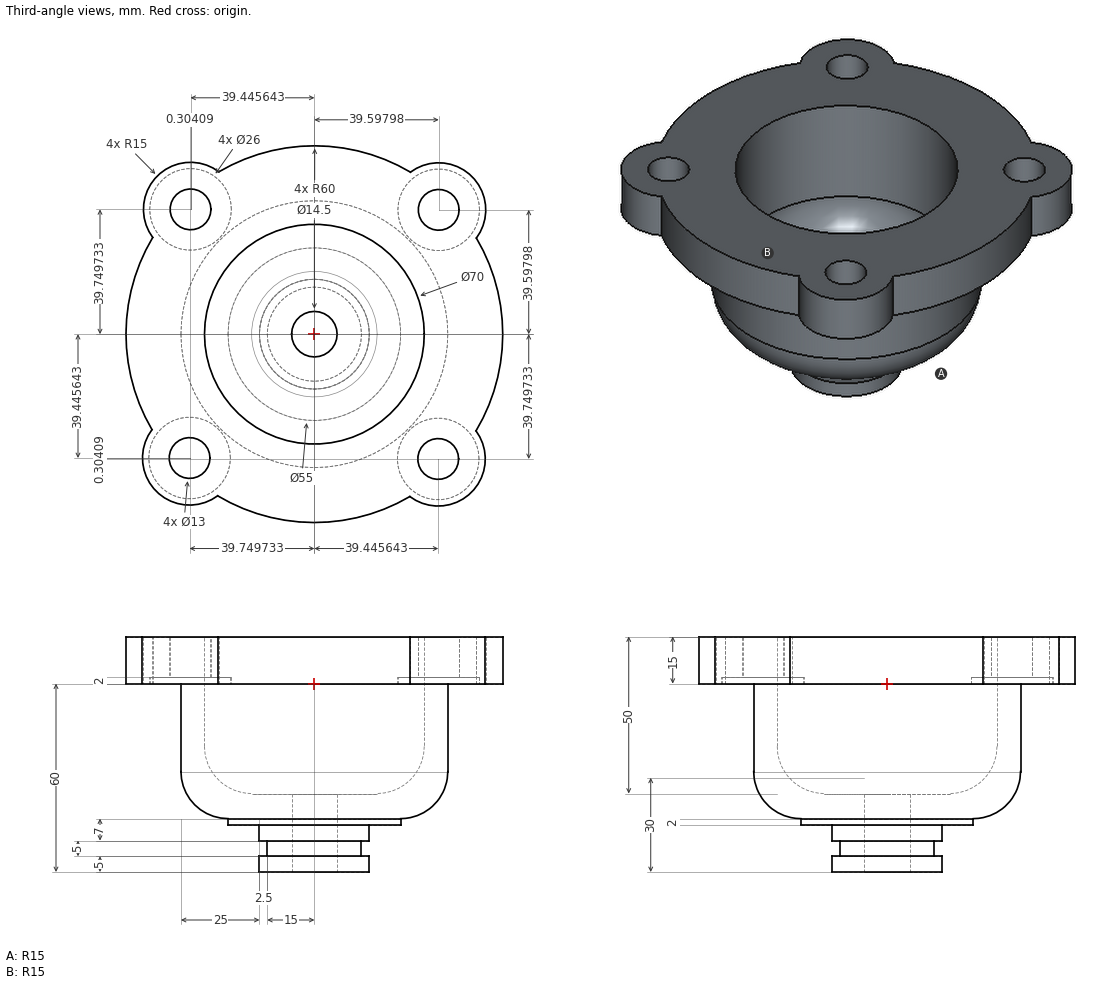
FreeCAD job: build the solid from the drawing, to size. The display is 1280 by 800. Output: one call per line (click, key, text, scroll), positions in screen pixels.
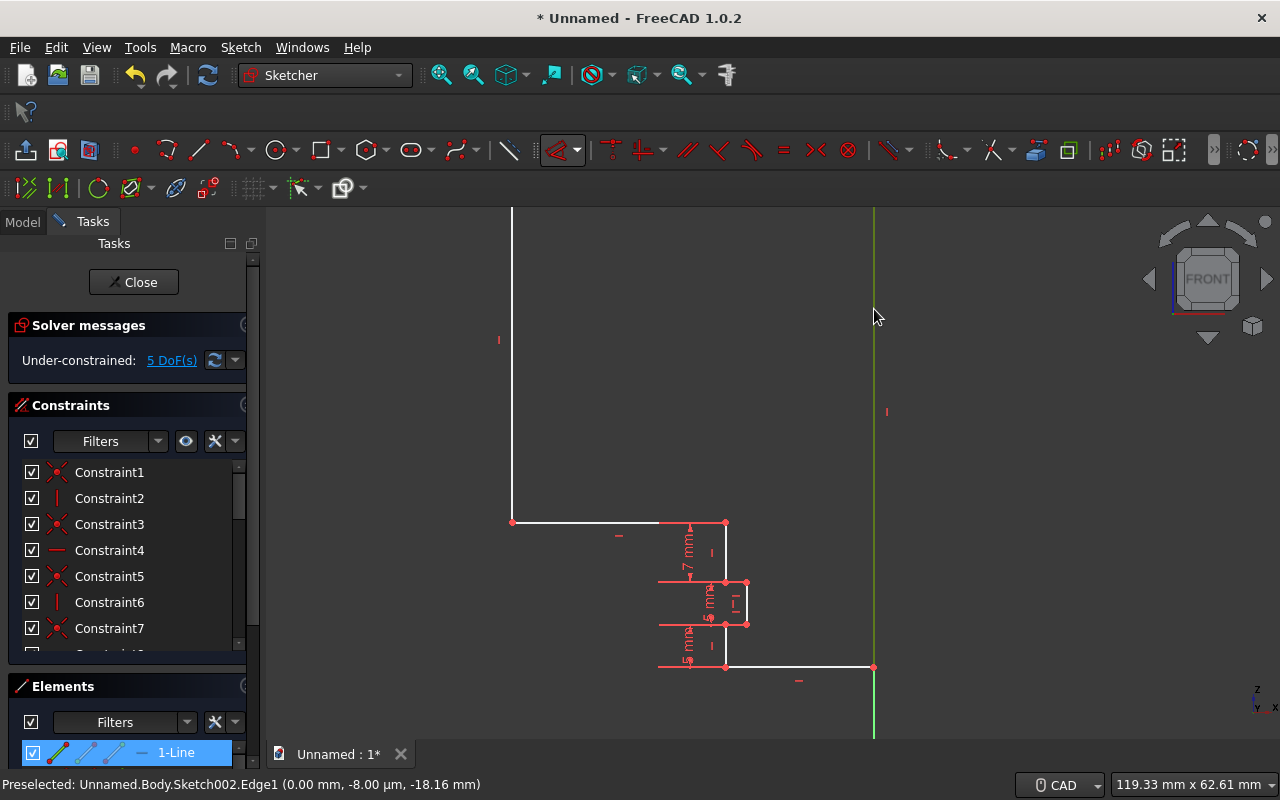
key(i)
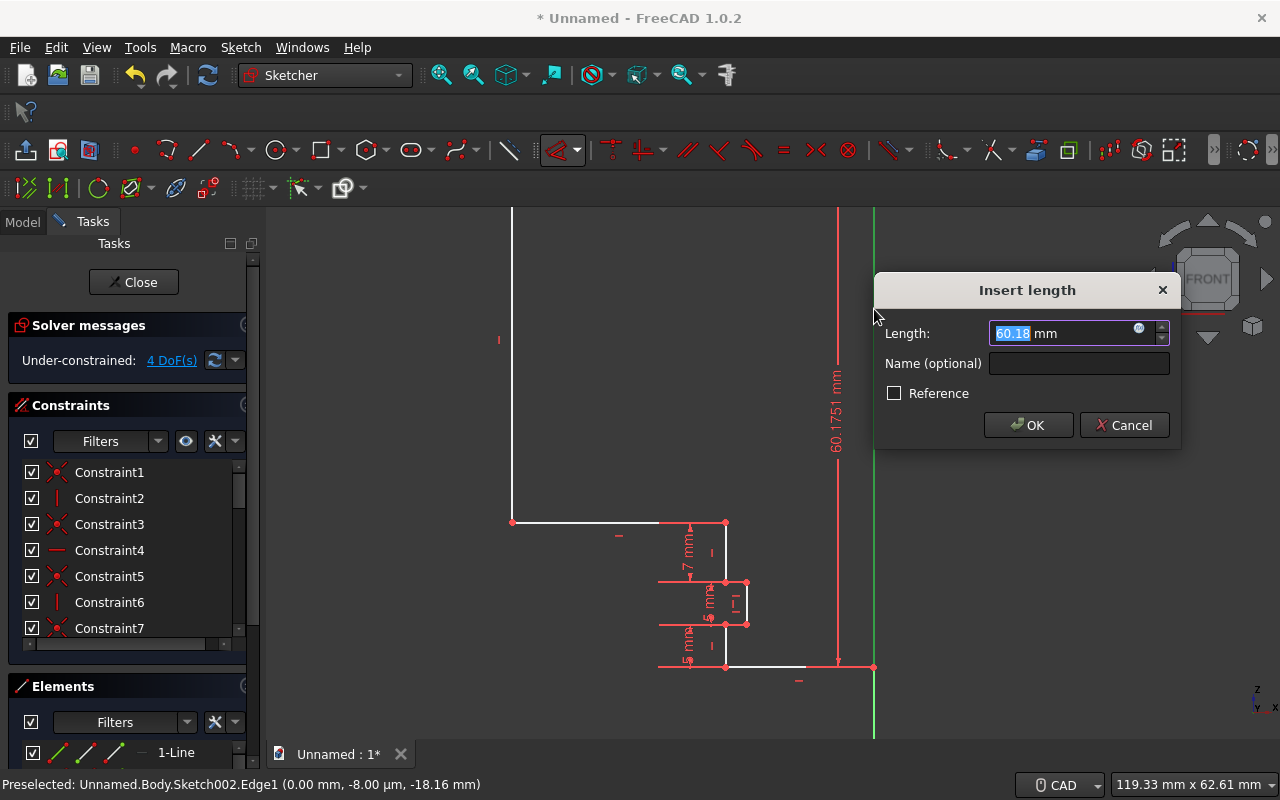
text(60)
key(Return)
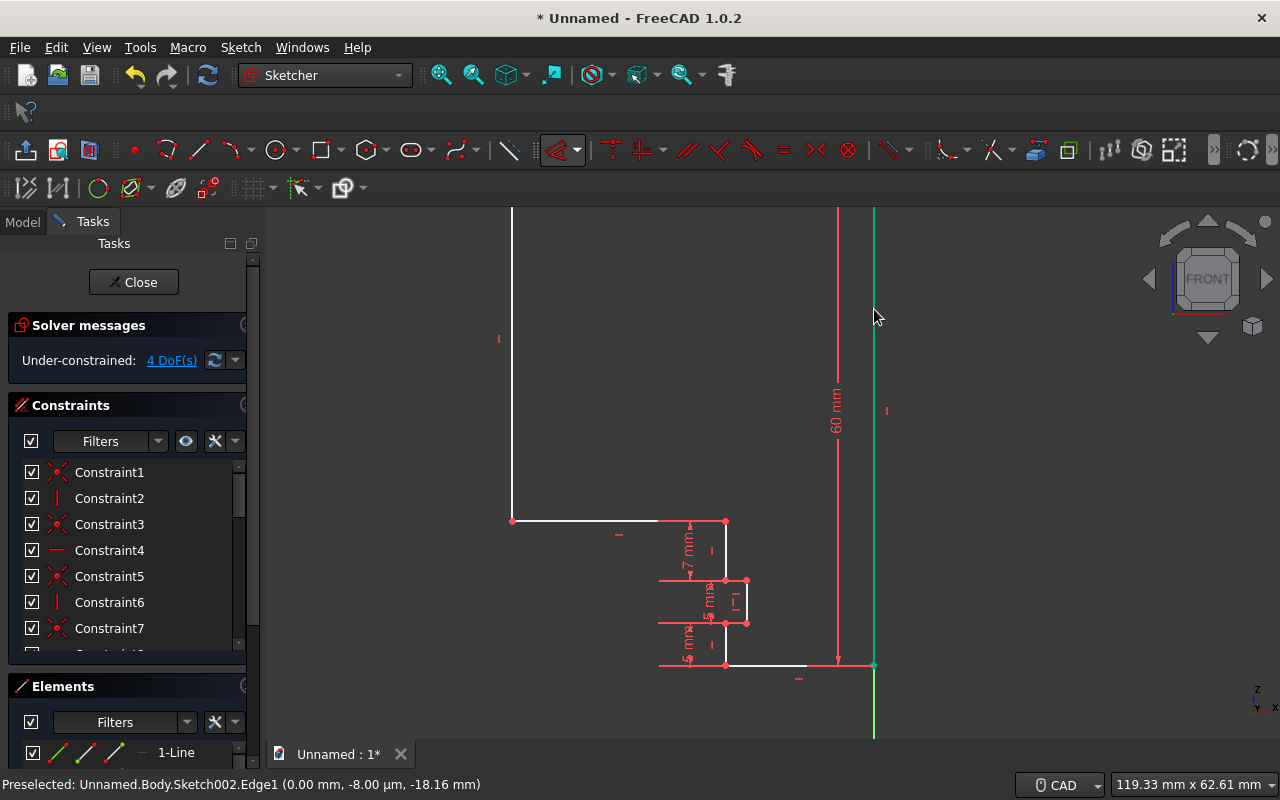
click(662, 521)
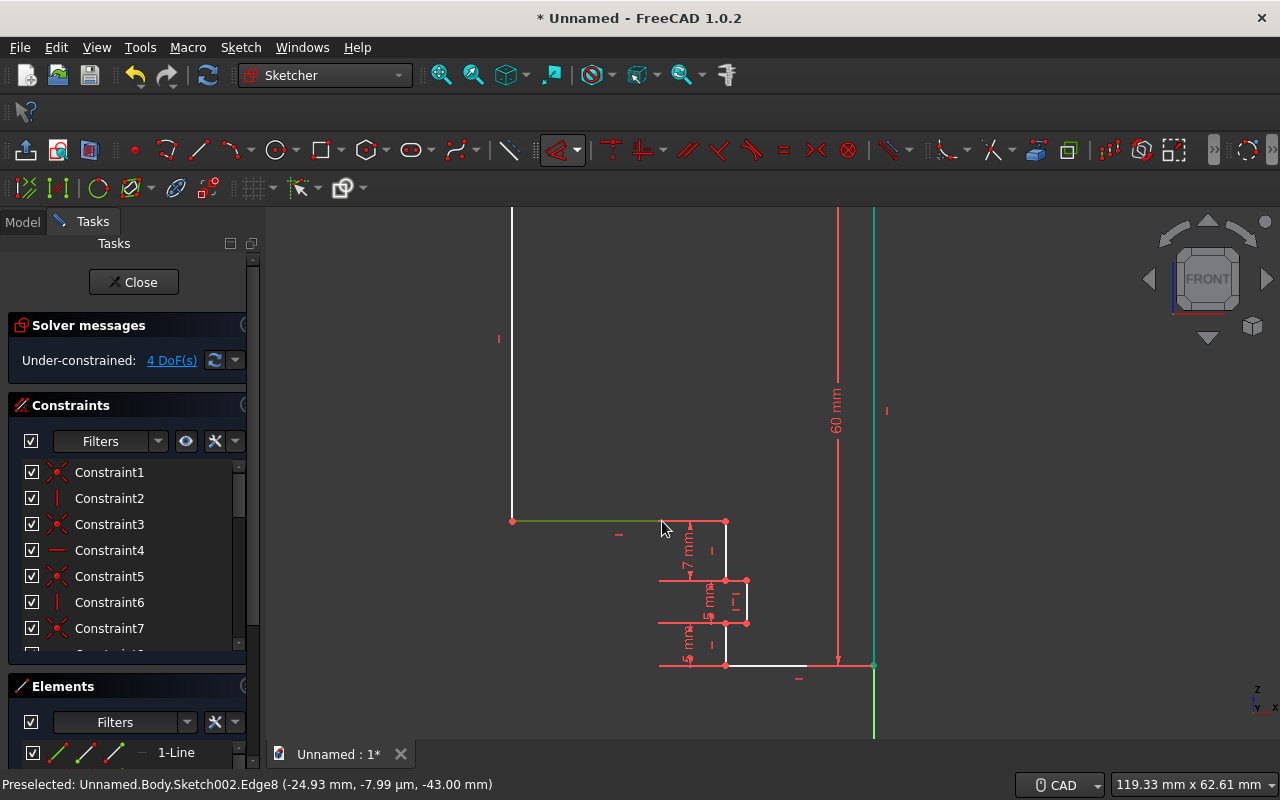
click(580, 150)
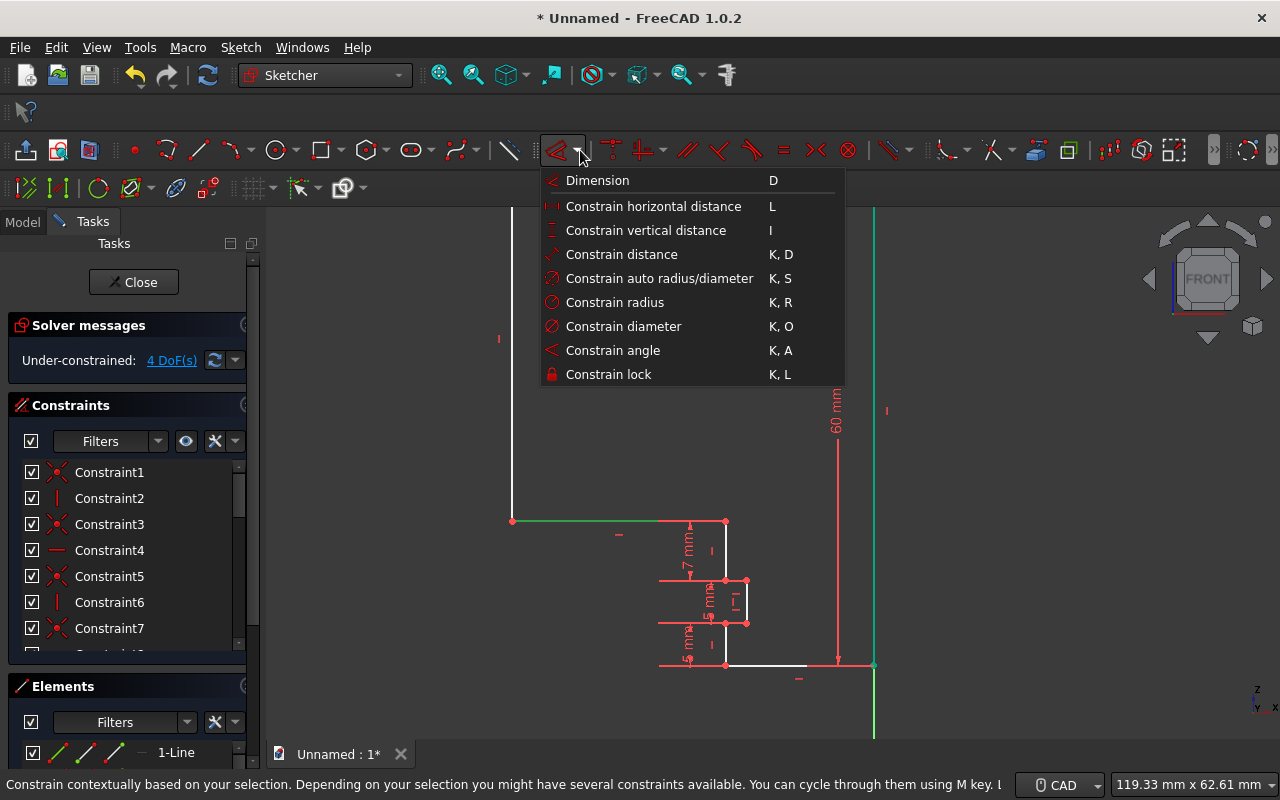
click(693, 206)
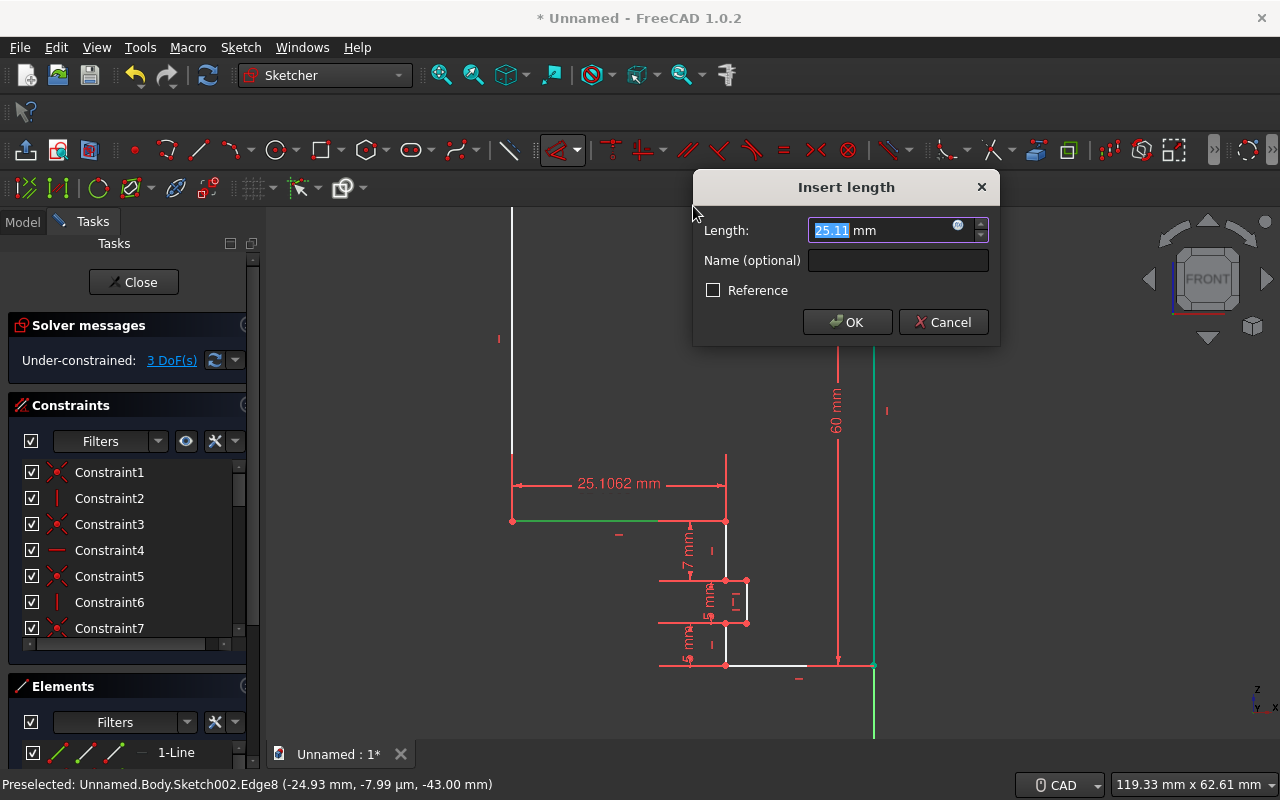
text(25)
key(Return)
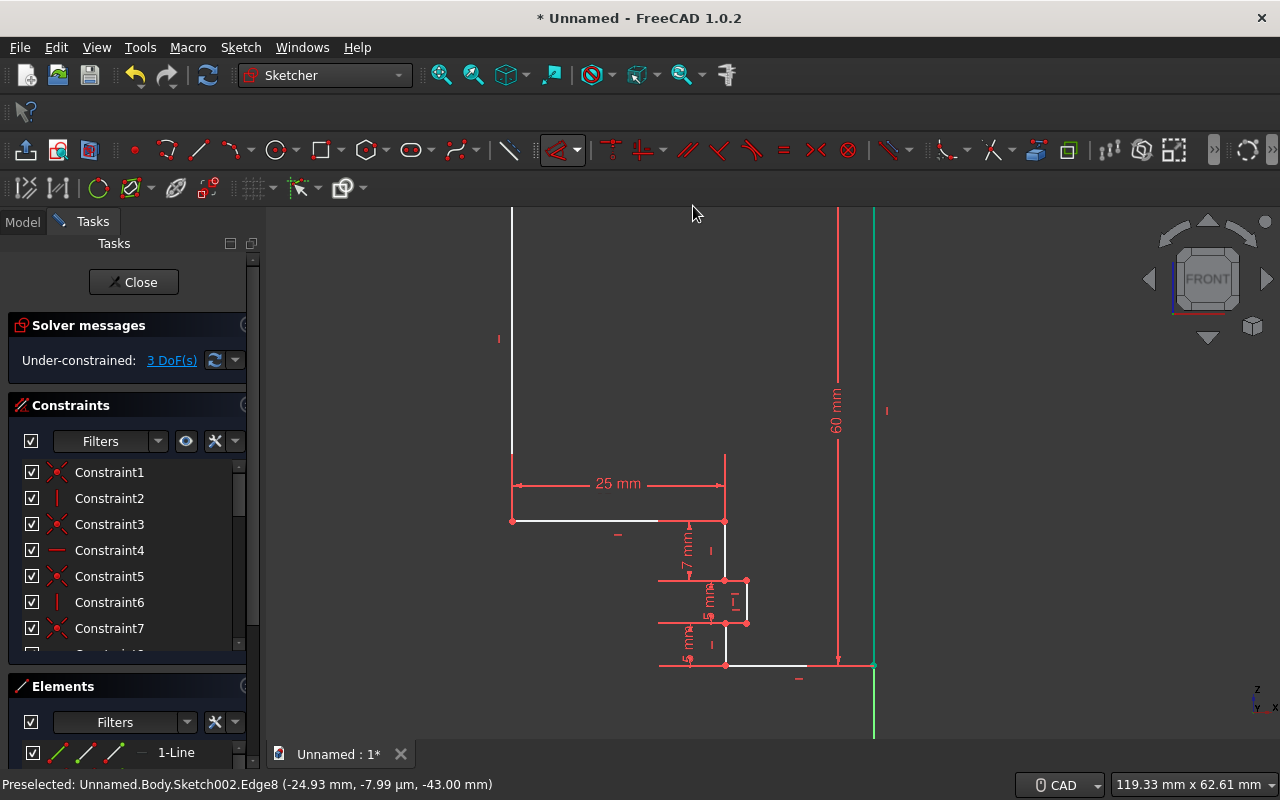
scroll(736, 623, up, 4)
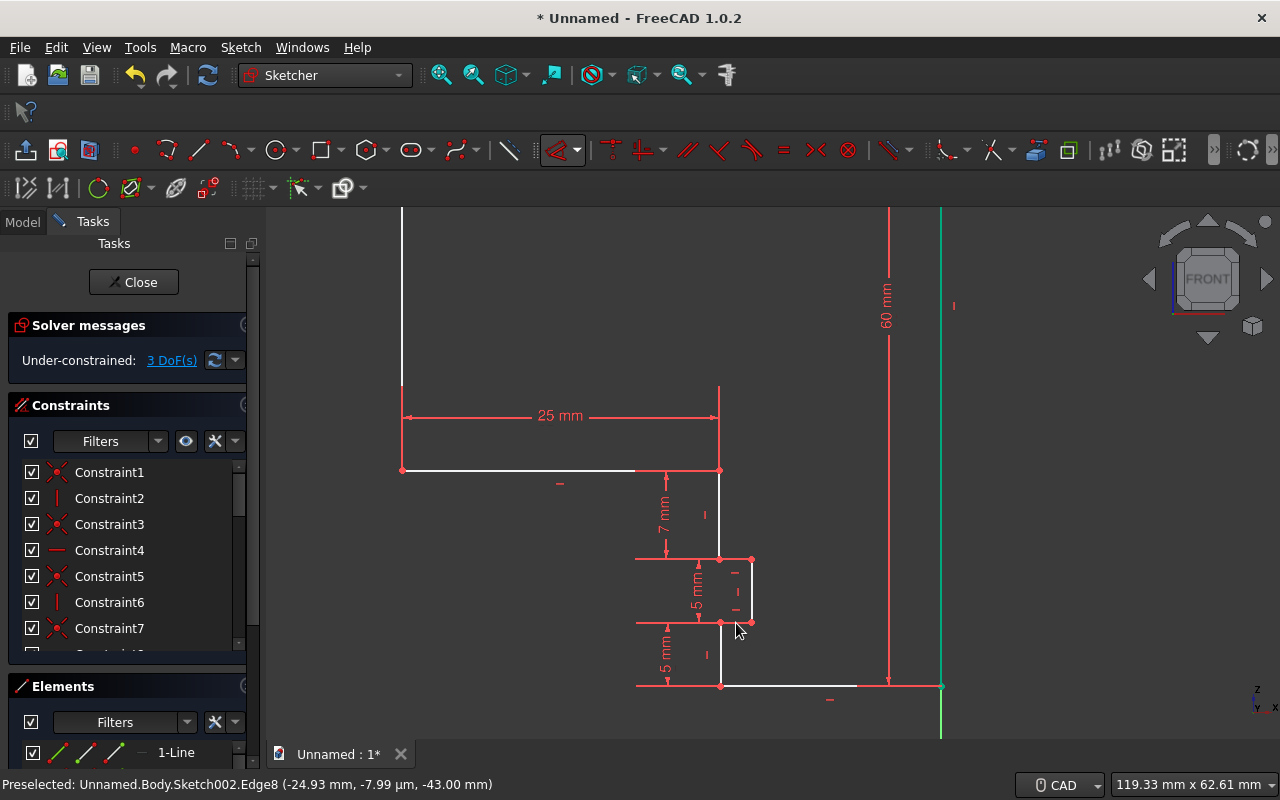
click(736, 622)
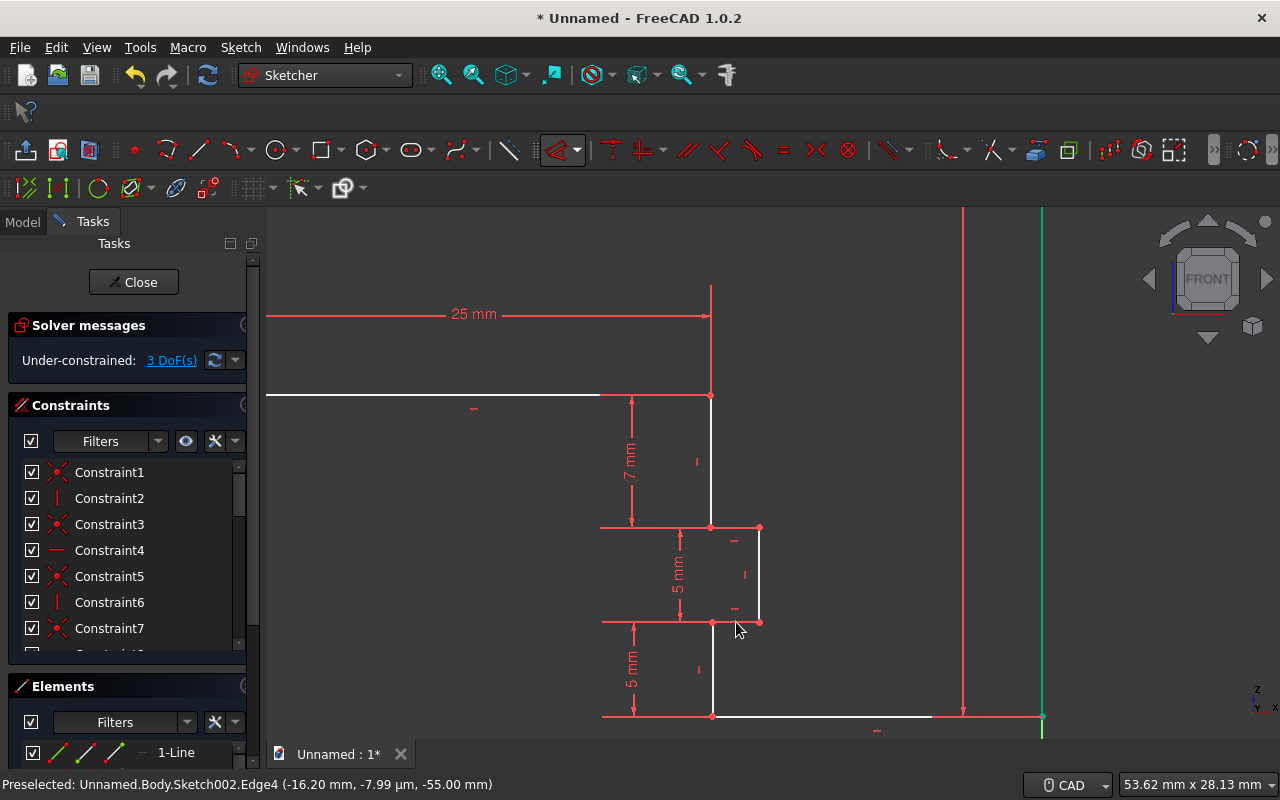
key(l)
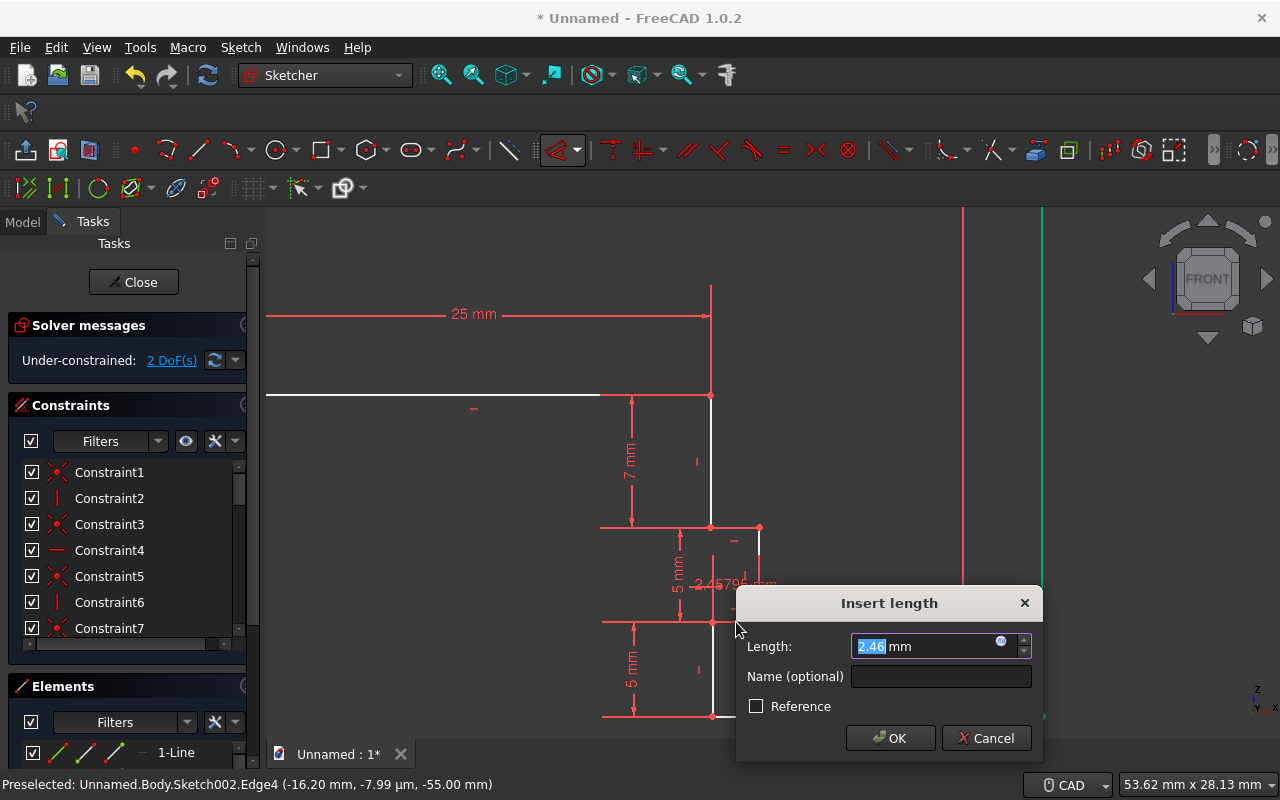
text(2.5)
key(Return)